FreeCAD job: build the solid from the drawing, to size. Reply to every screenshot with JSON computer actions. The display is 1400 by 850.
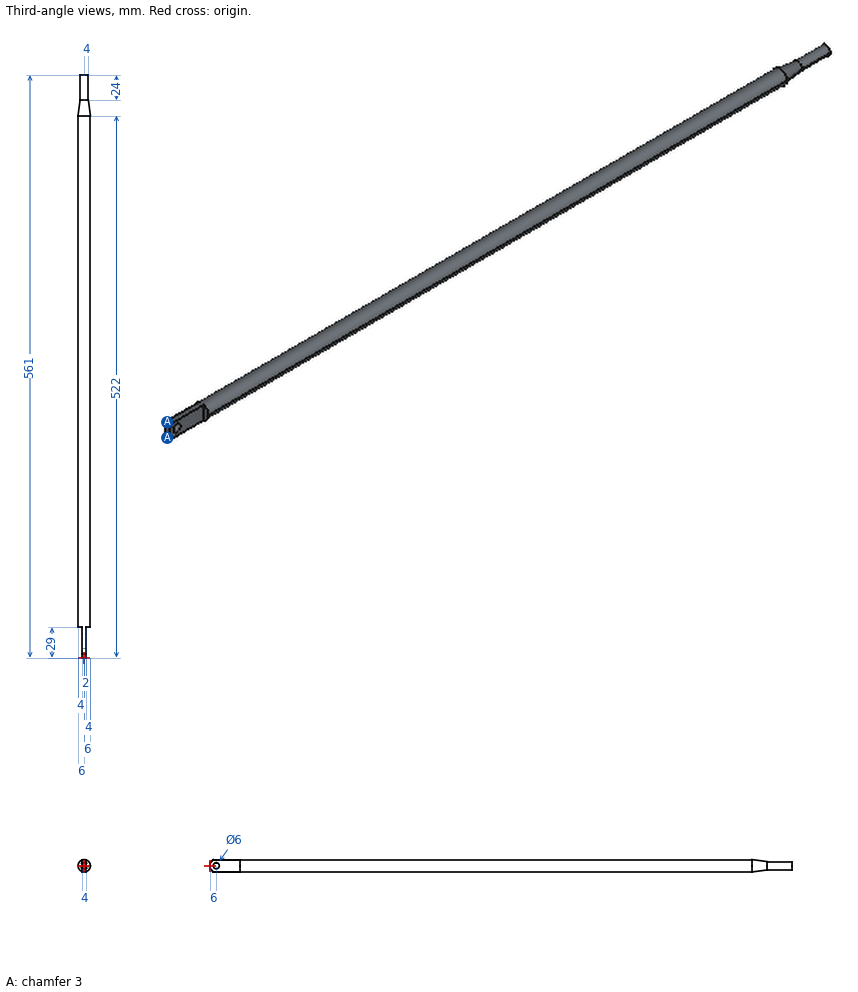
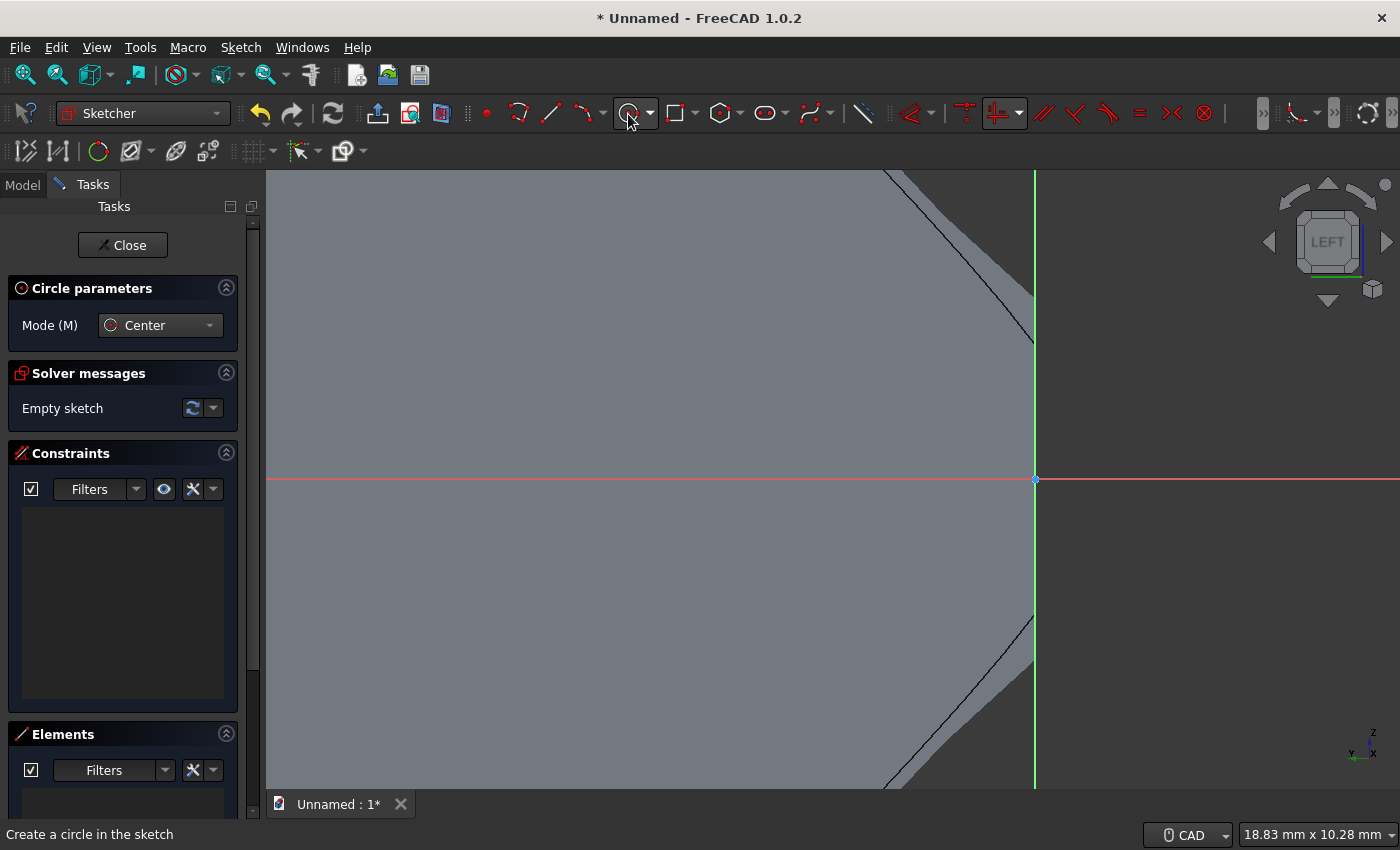
{"action": "left_click", "coordinate": [674, 479]}
{"action": "left_click", "coordinate": [802, 352]}
{"action": "key", "text": "Escape"}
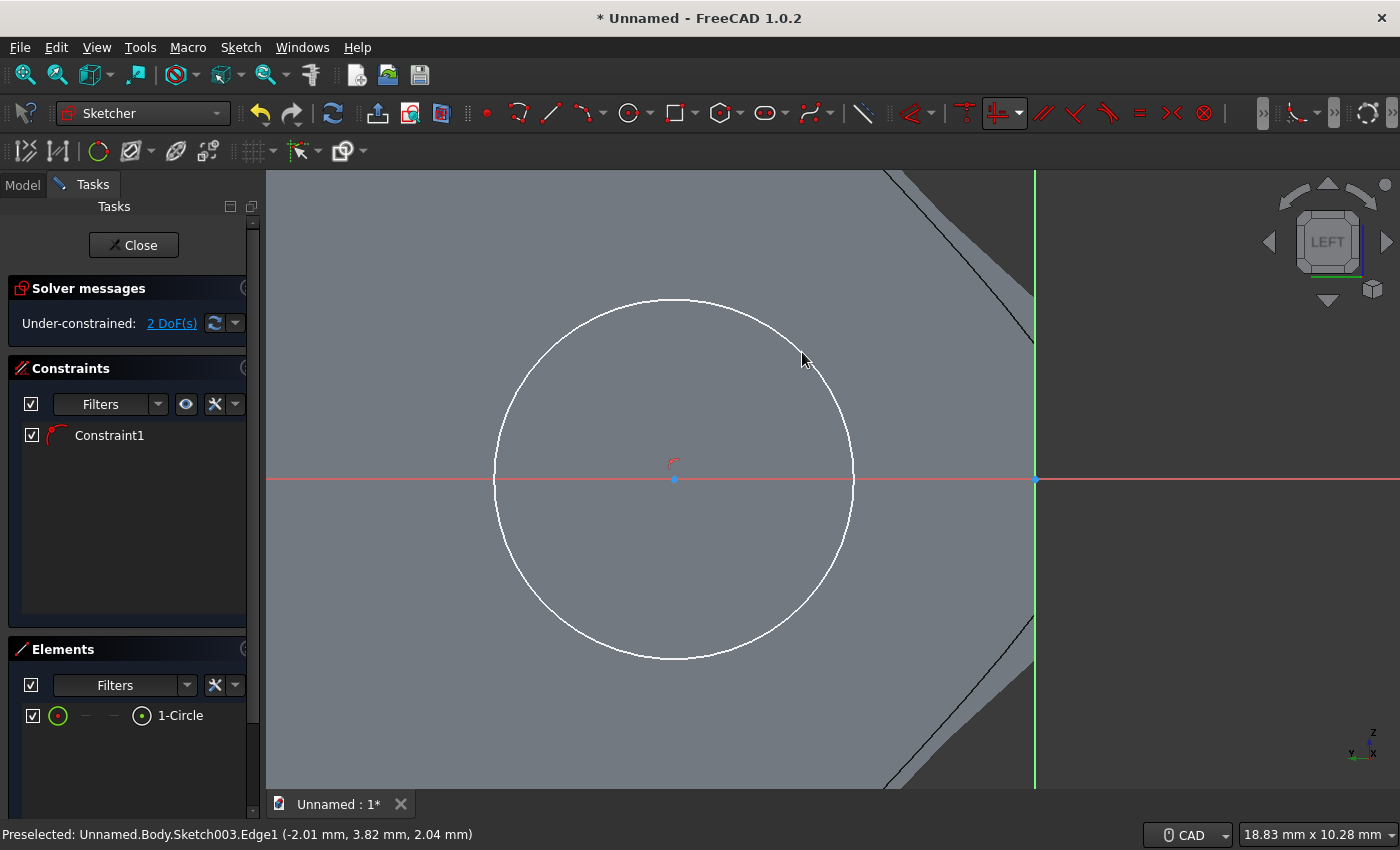
{"action": "left_click", "coordinate": [910, 114]}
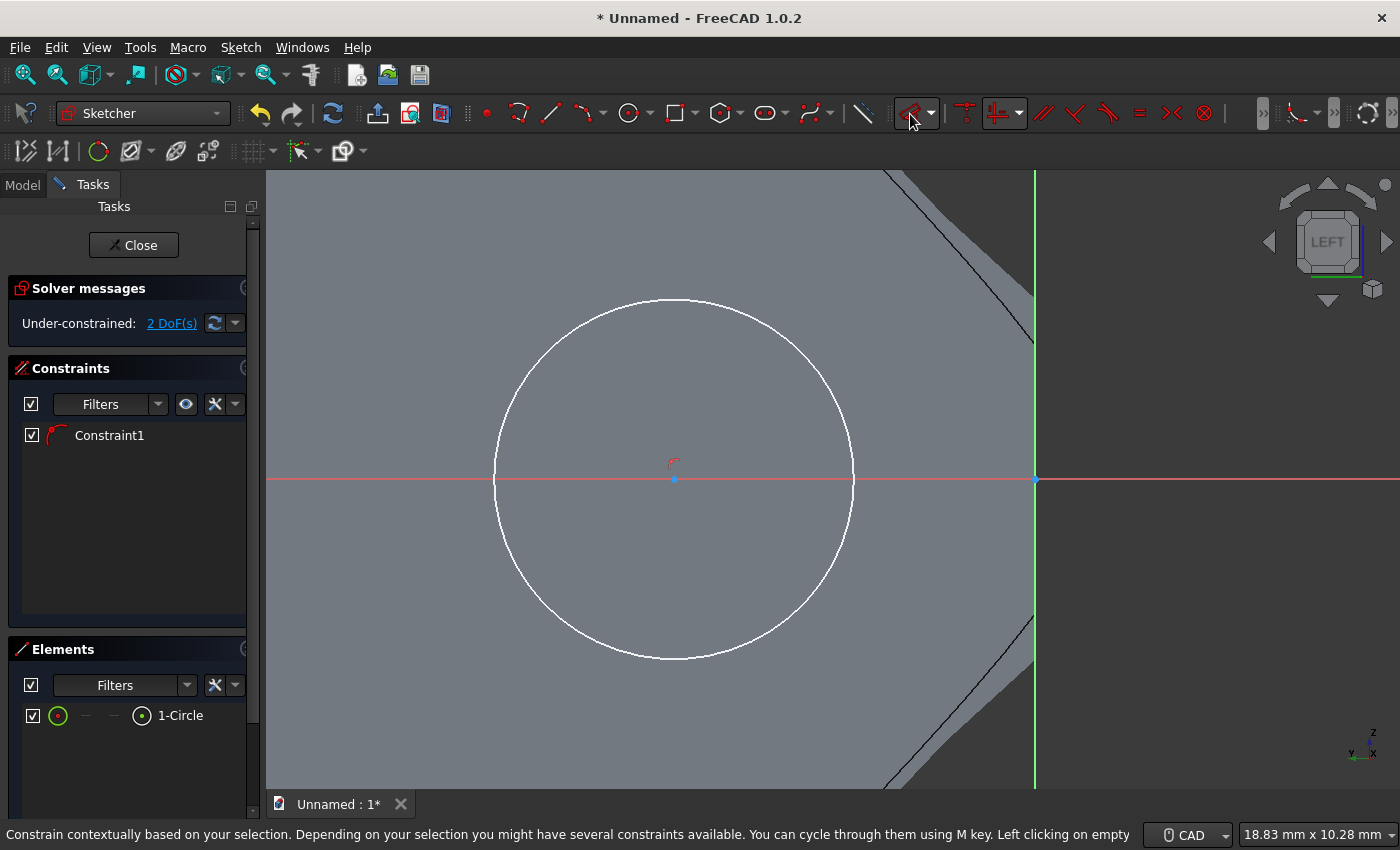
{"action": "left_click", "coordinate": [801, 352]}
{"action": "left_click", "coordinate": [824, 329]}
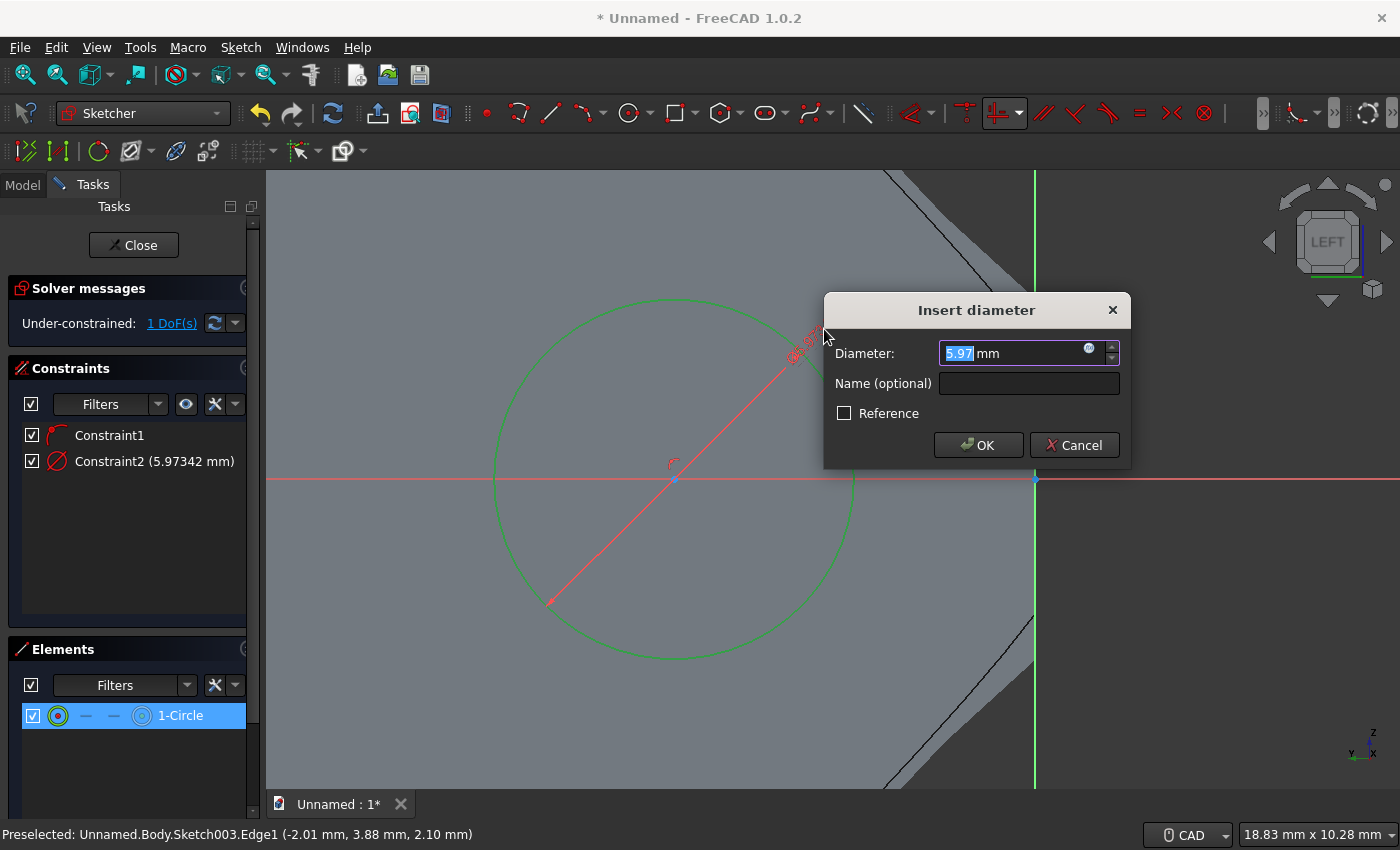
{"action": "type", "text": "6"}
{"action": "key", "text": "Return"}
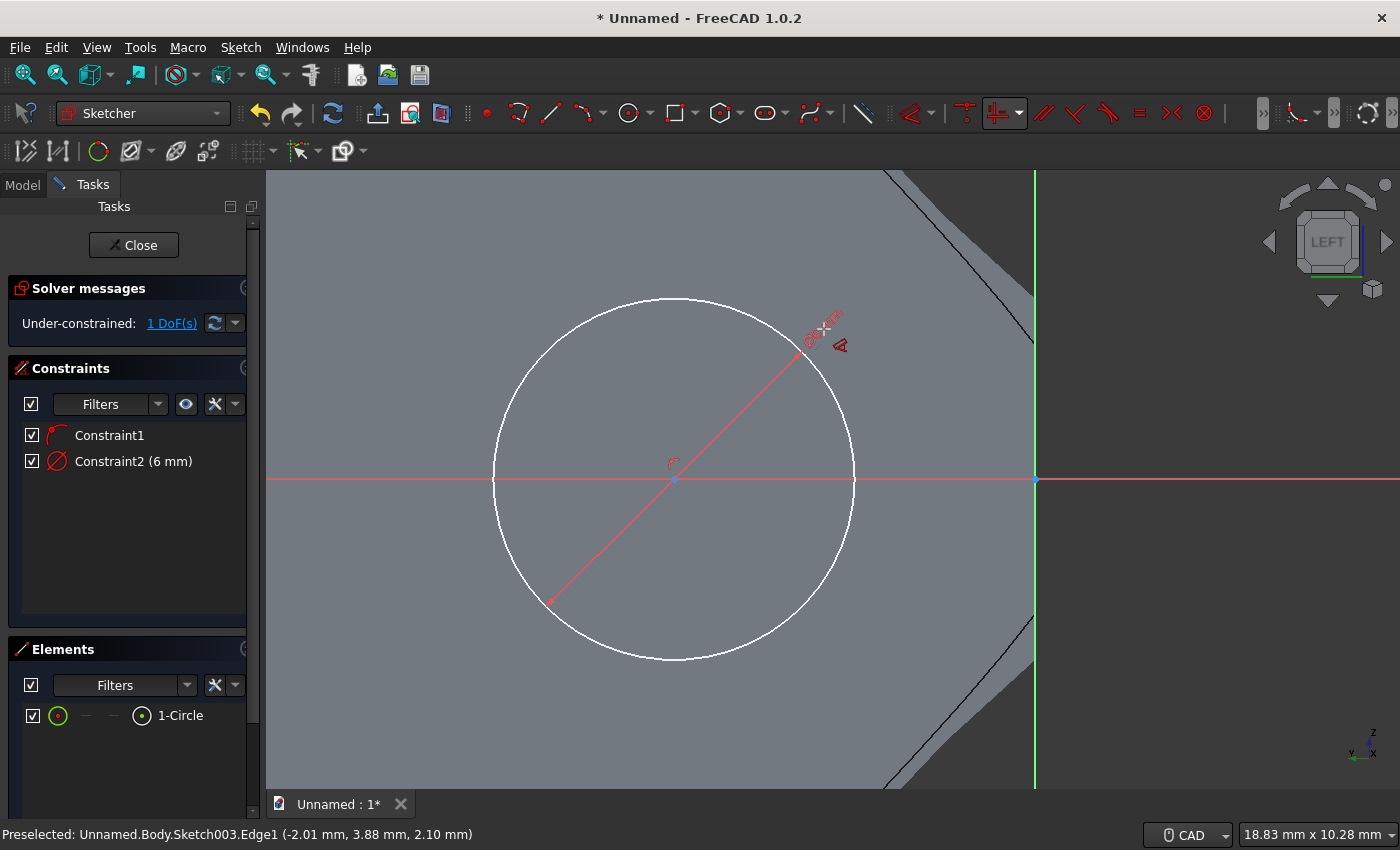
{"action": "left_click", "coordinate": [674, 479]}
{"action": "left_click", "coordinate": [771, 513]}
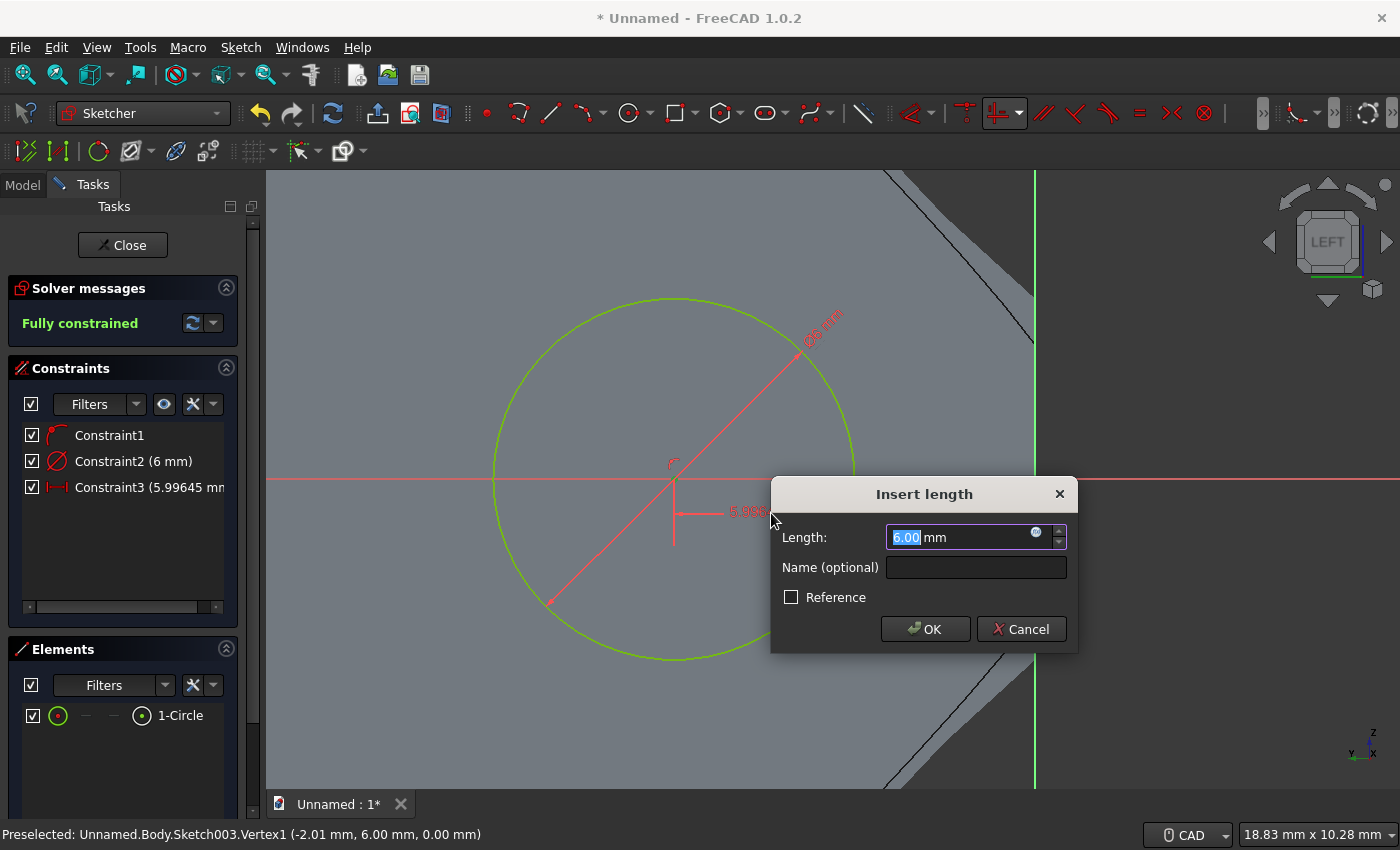
{"action": "type", "text": "6"}
{"action": "key", "text": "Return"}
{"action": "key", "text": "Escape"}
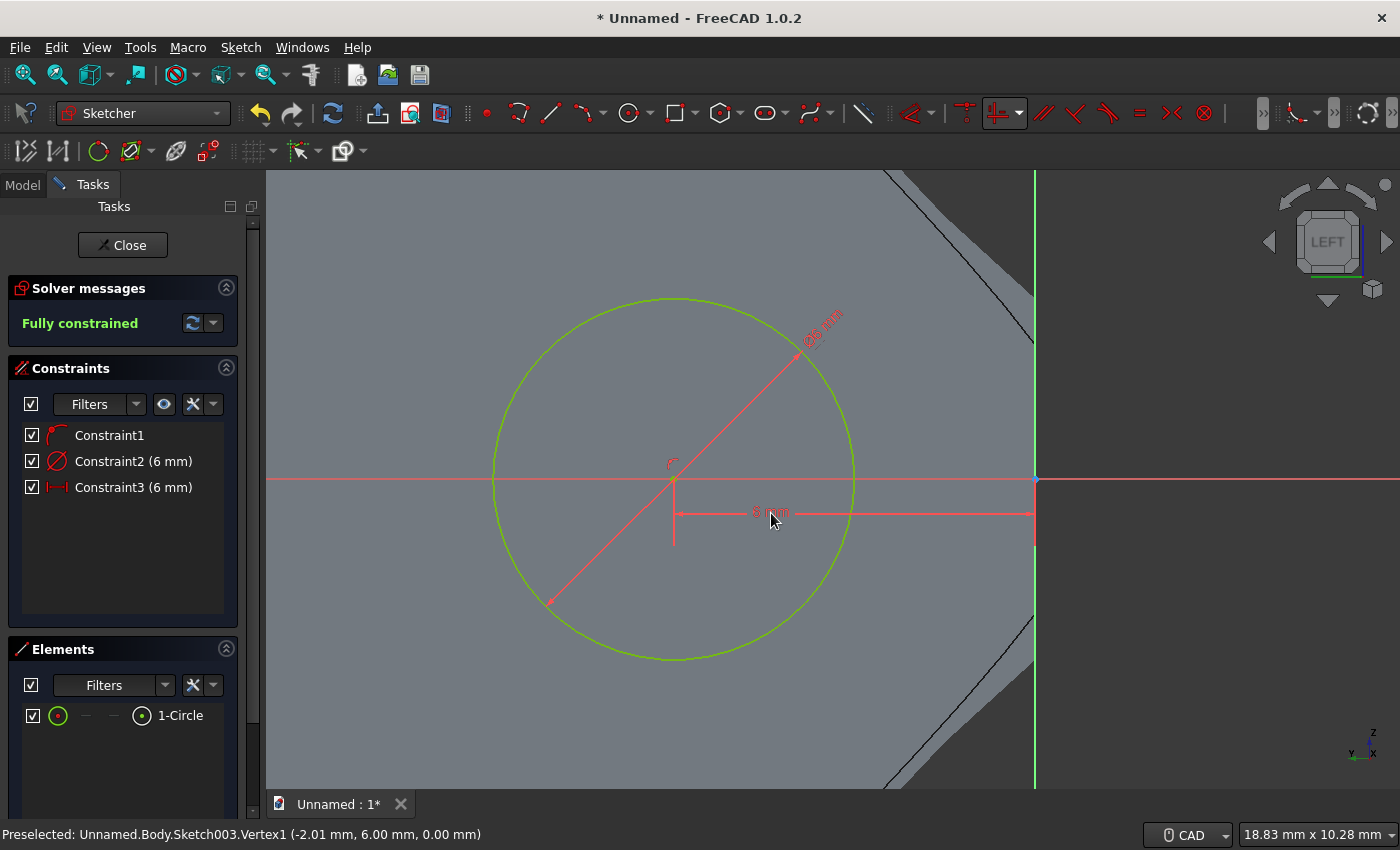
{"action": "left_click", "coordinate": [123, 245]}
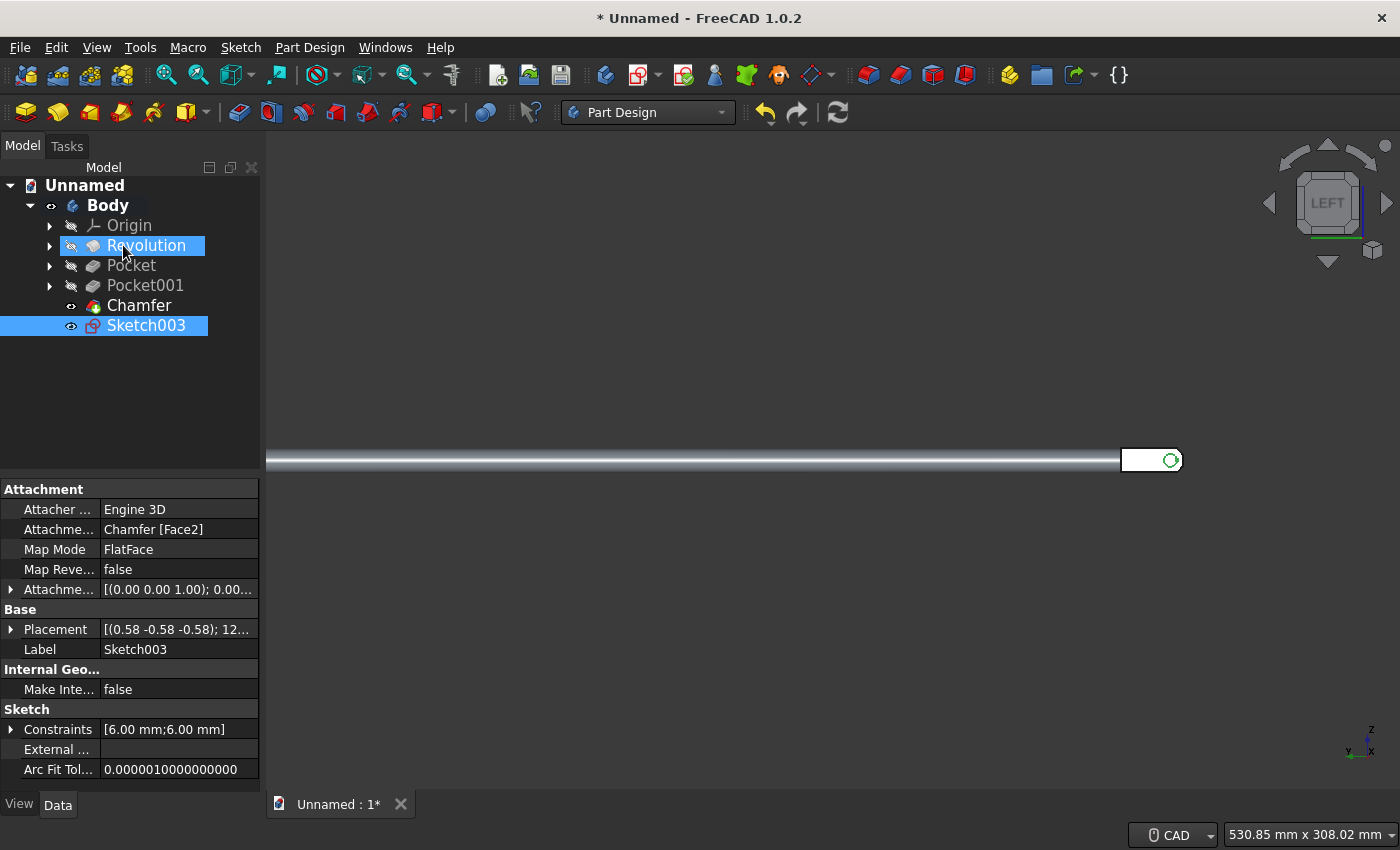
{"action": "left_click", "coordinate": [240, 112]}